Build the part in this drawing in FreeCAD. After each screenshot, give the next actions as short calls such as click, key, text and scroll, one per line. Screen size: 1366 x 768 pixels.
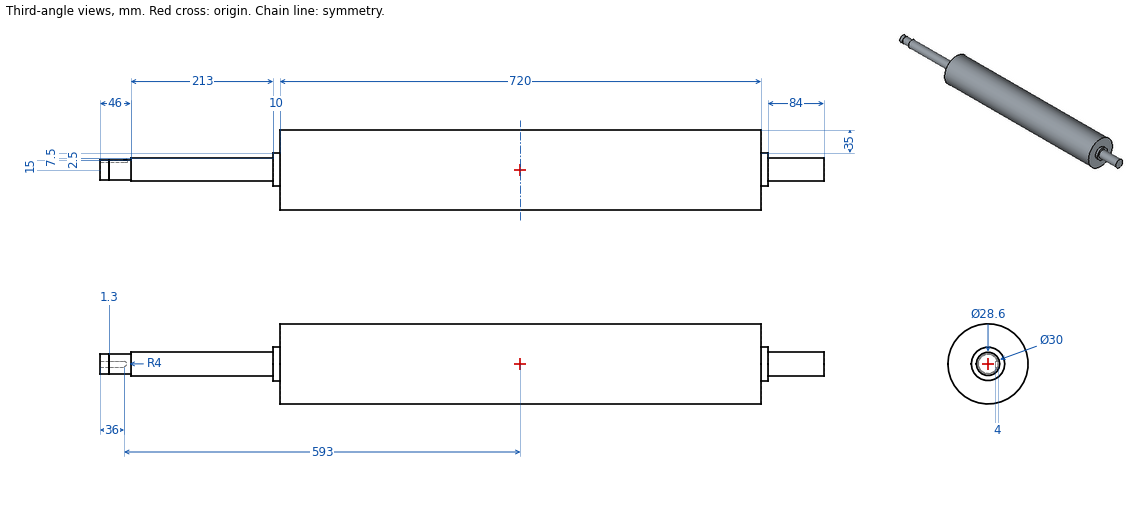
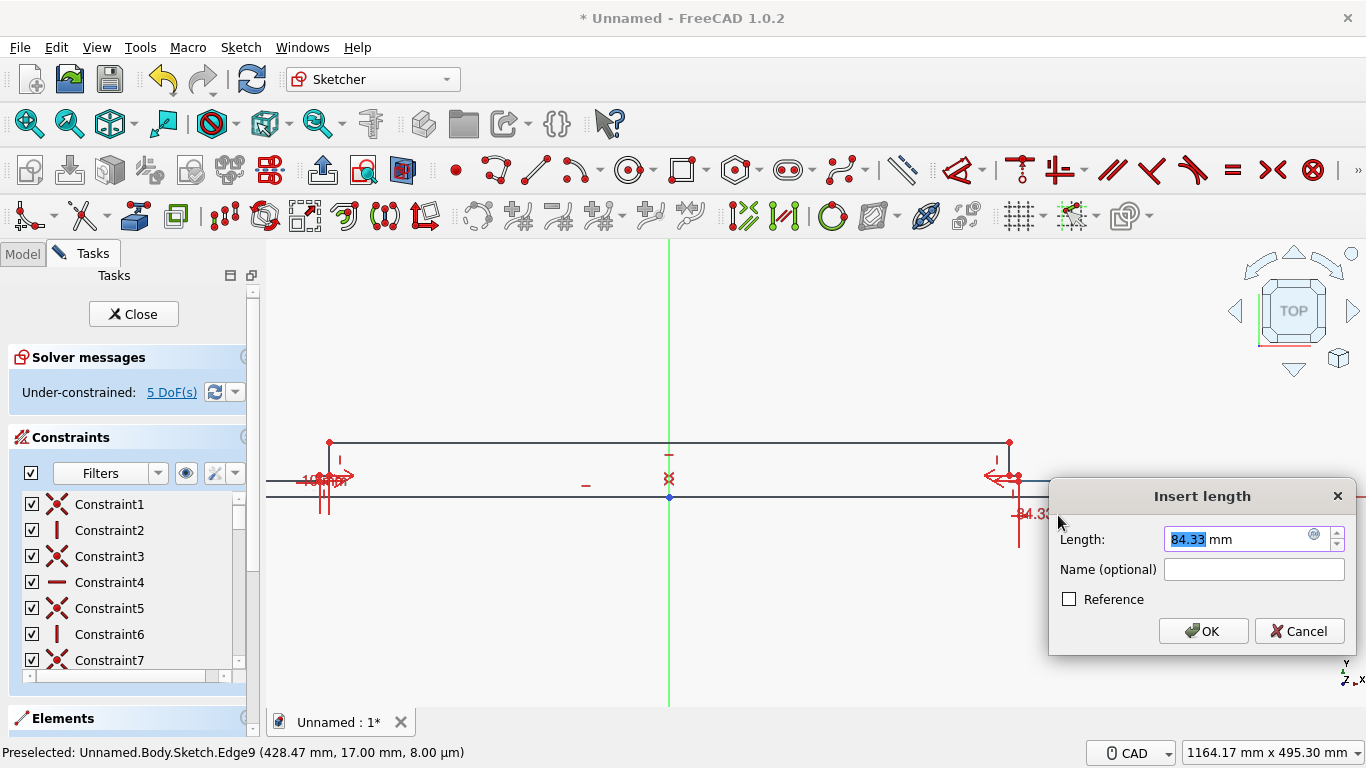
text(84)
key(Return)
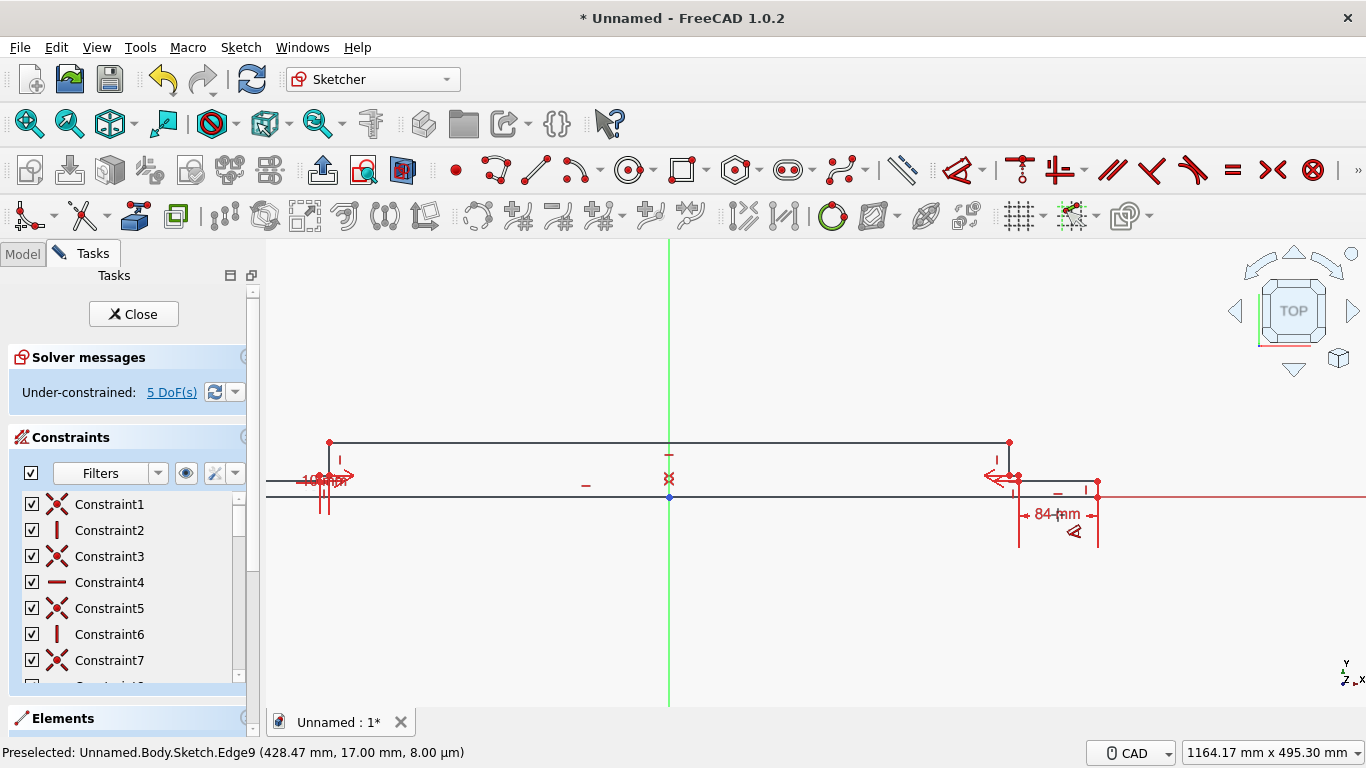
scroll(1009, 466, up, 2)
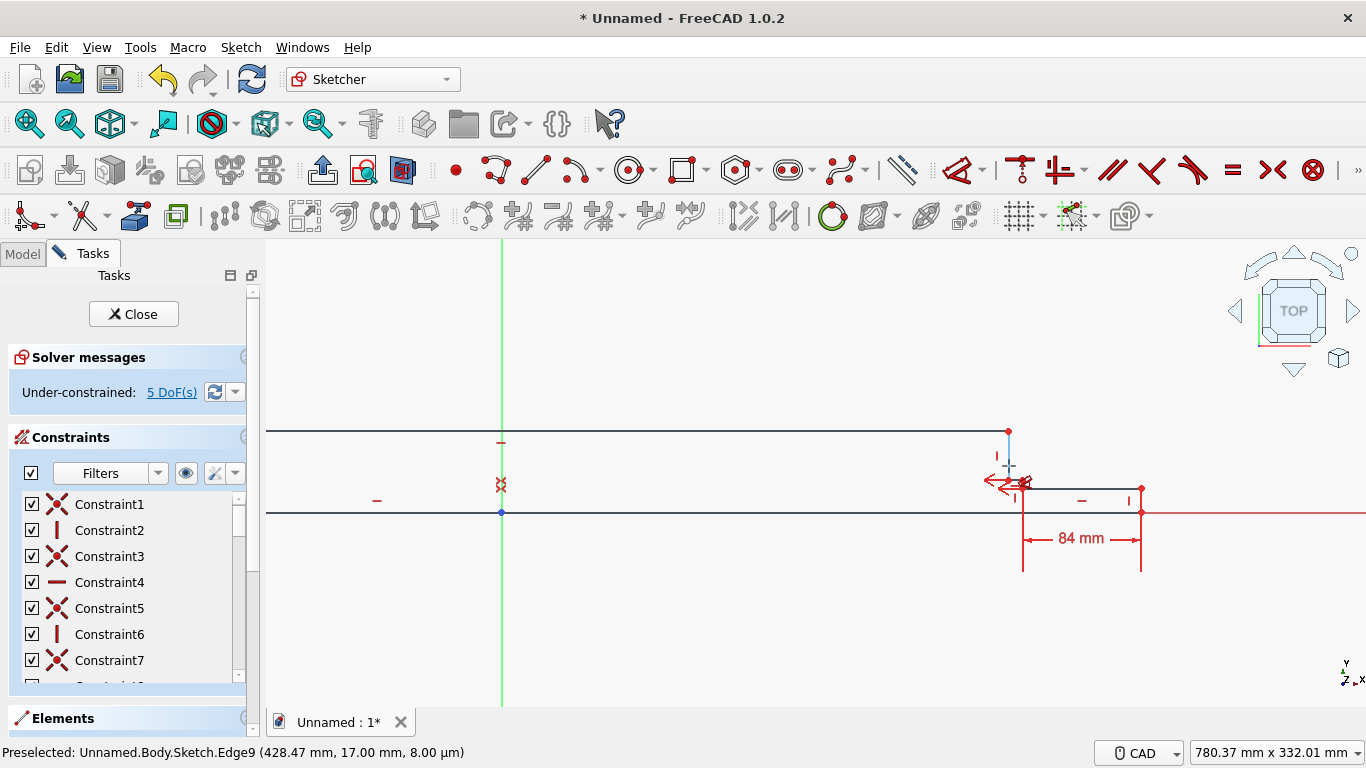
click(1009, 465)
click(1043, 456)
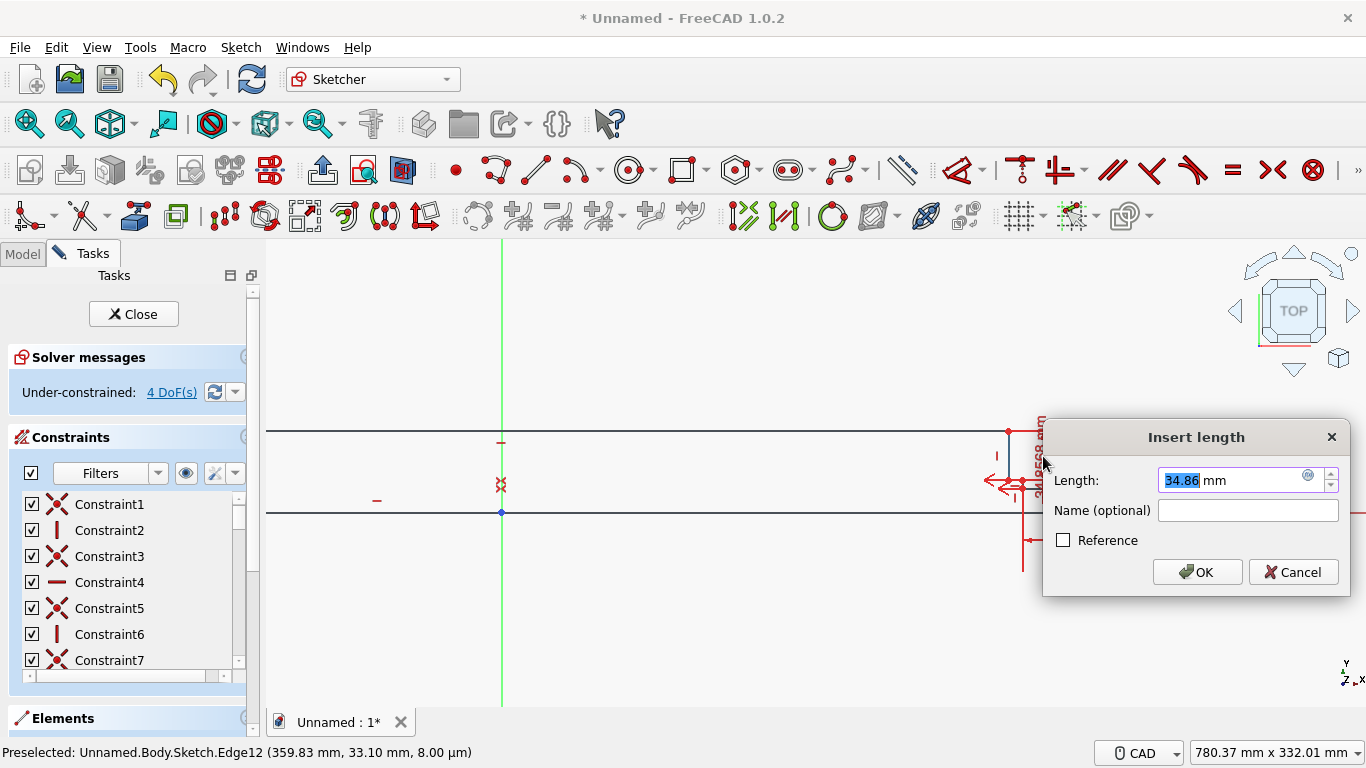
text(35)
key(Return)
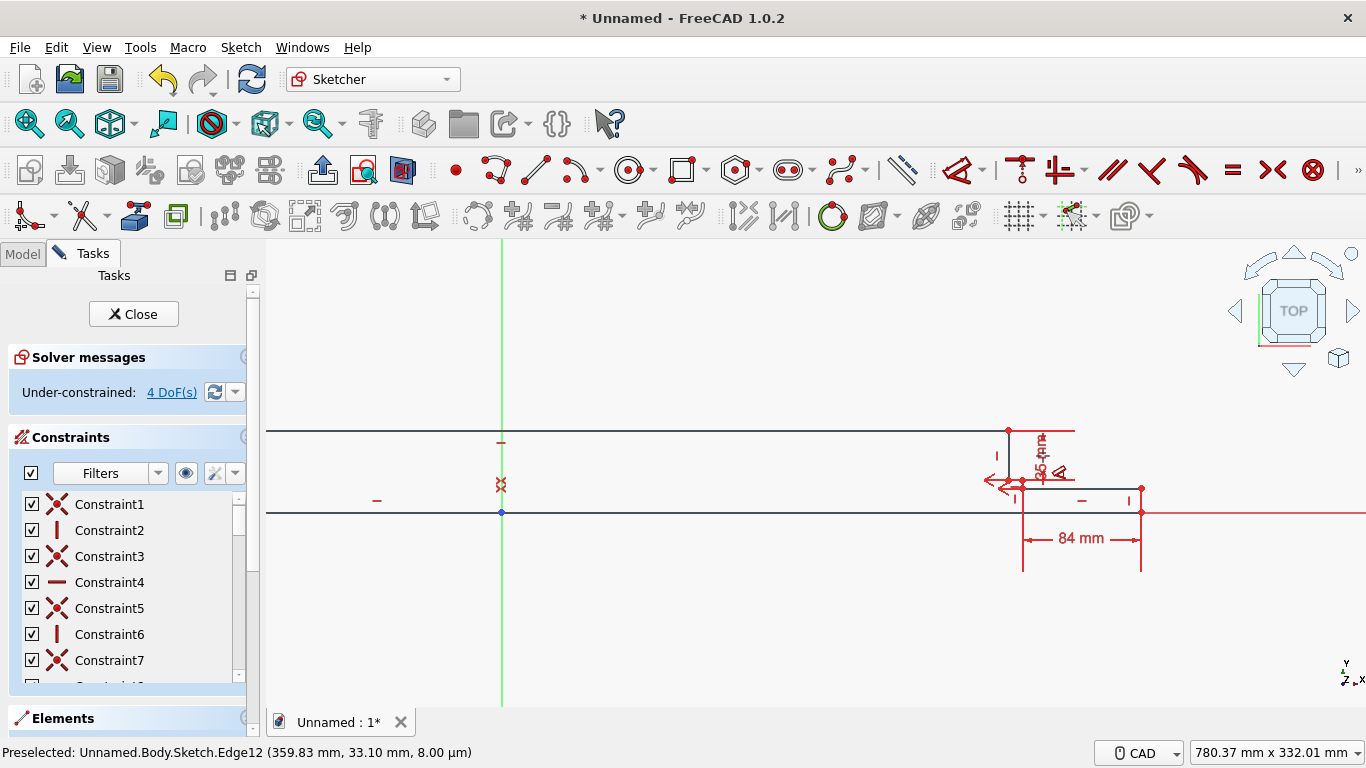
scroll(1049, 475, down, 4)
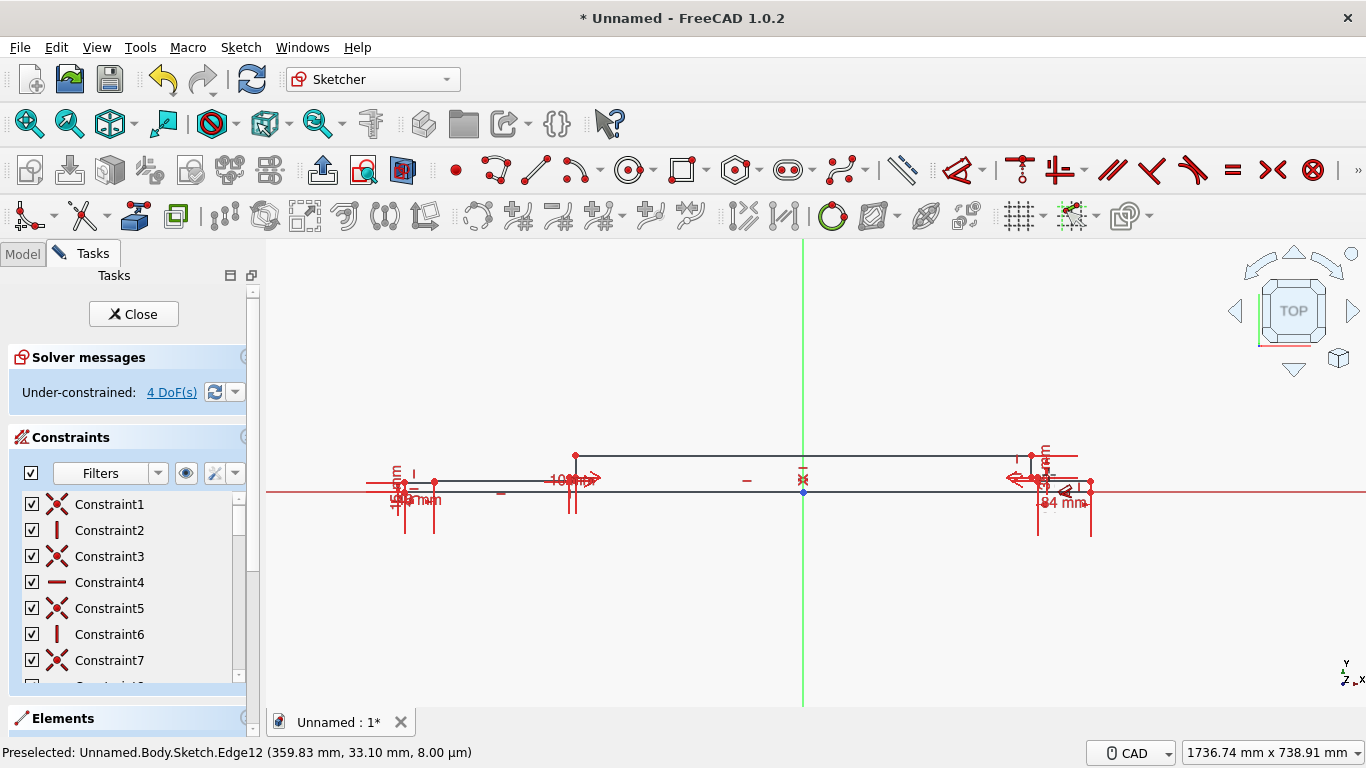
scroll(569, 480, up, 11)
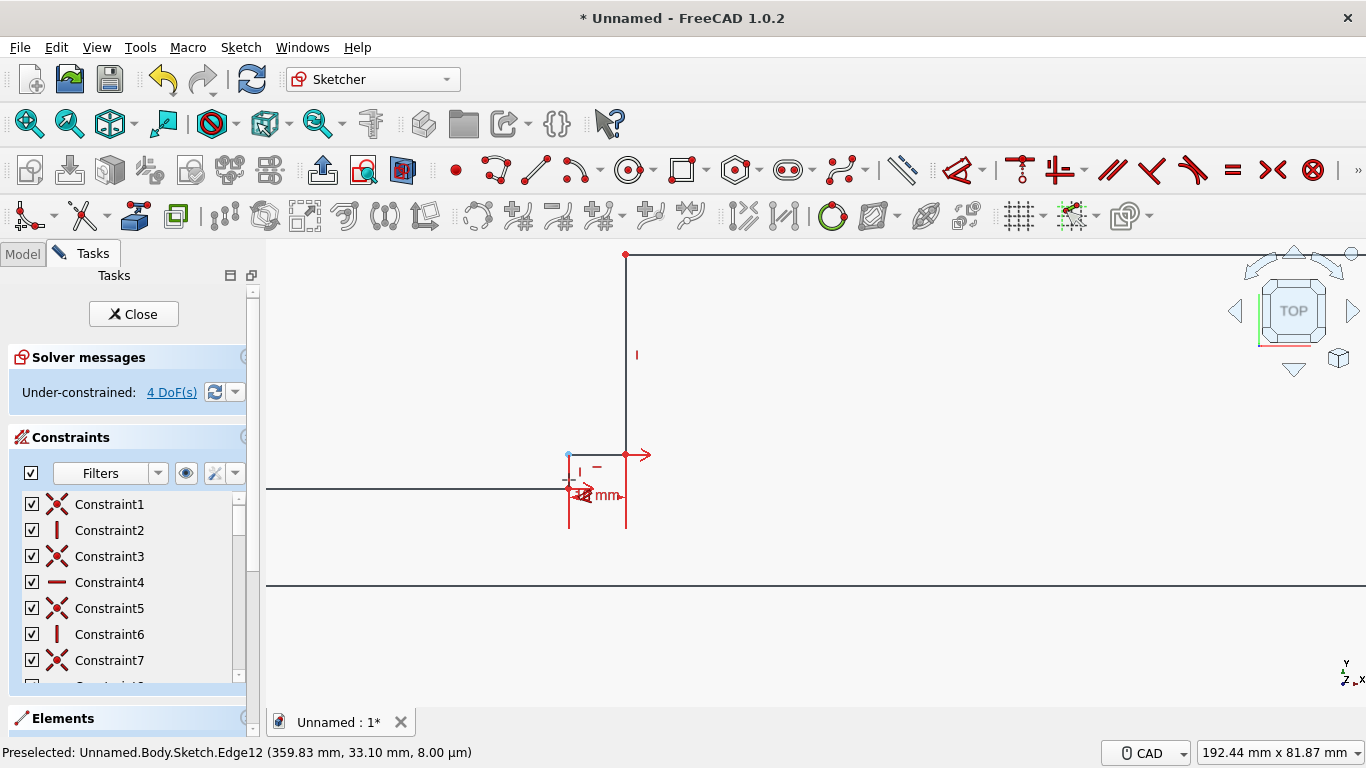
click(569, 472)
click(535, 472)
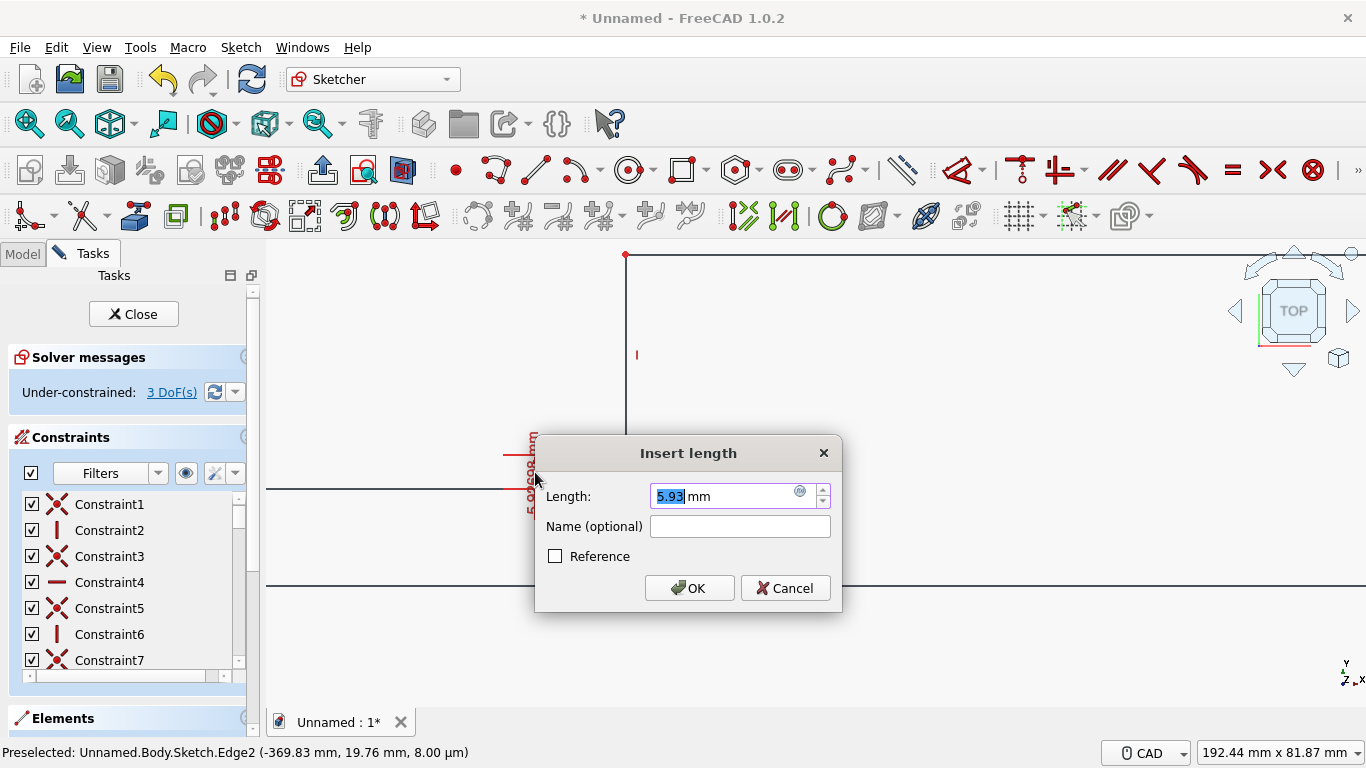
text(7.5)
key(Return)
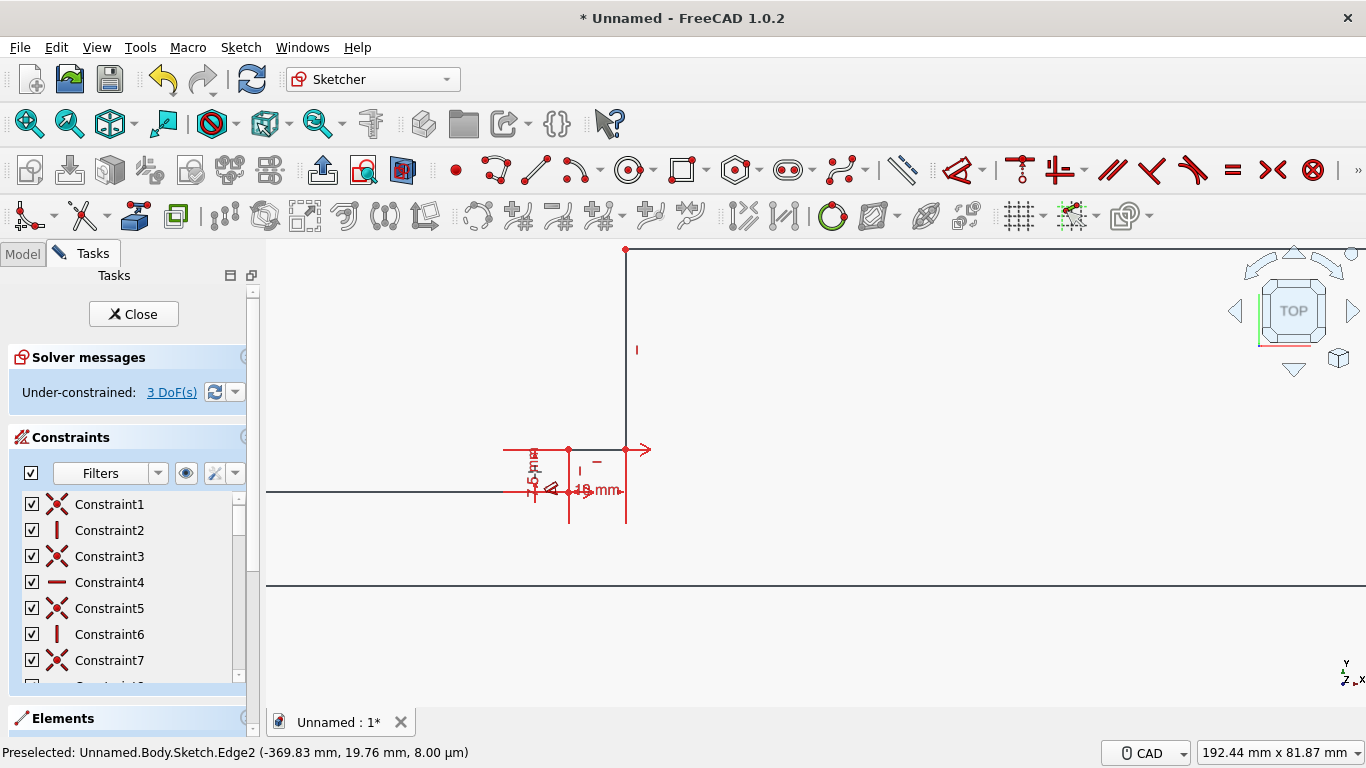
scroll(569, 480, down, 11)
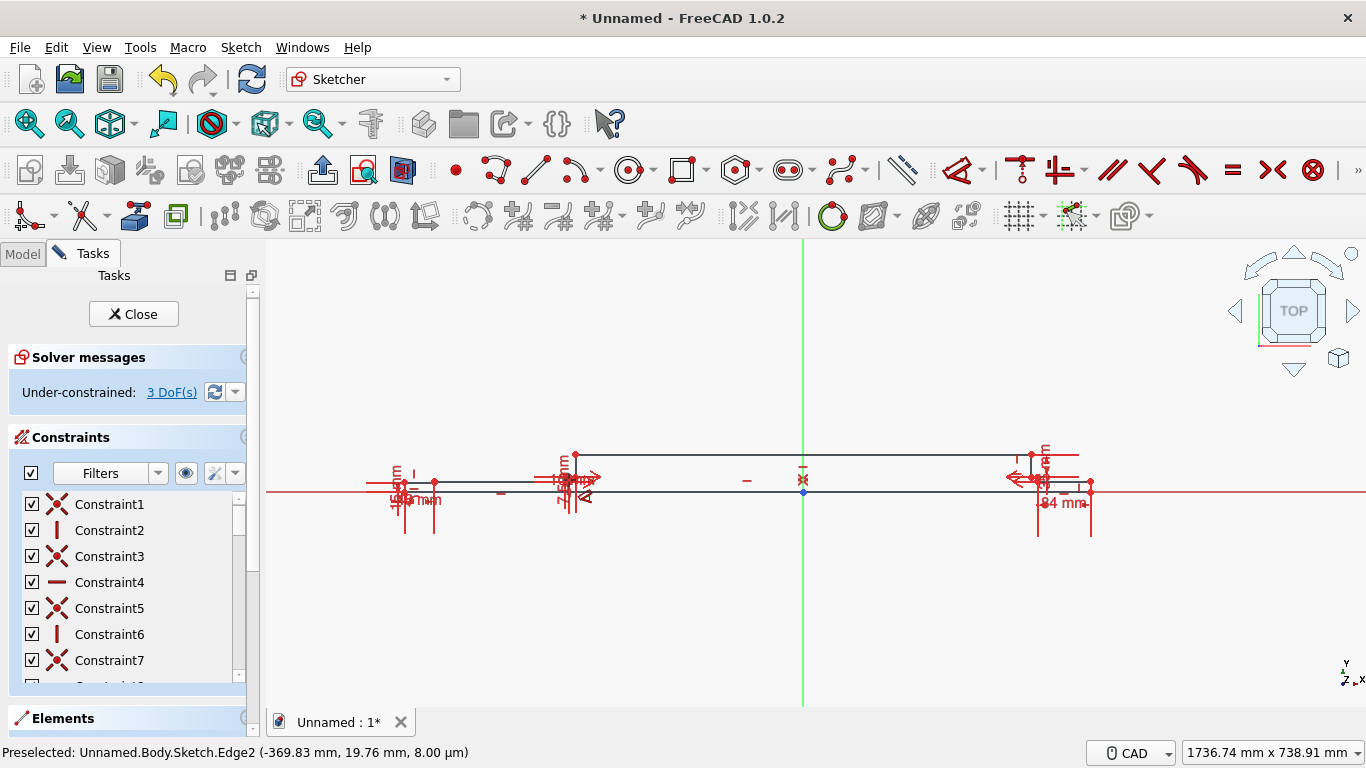
scroll(542, 482, up, 2)